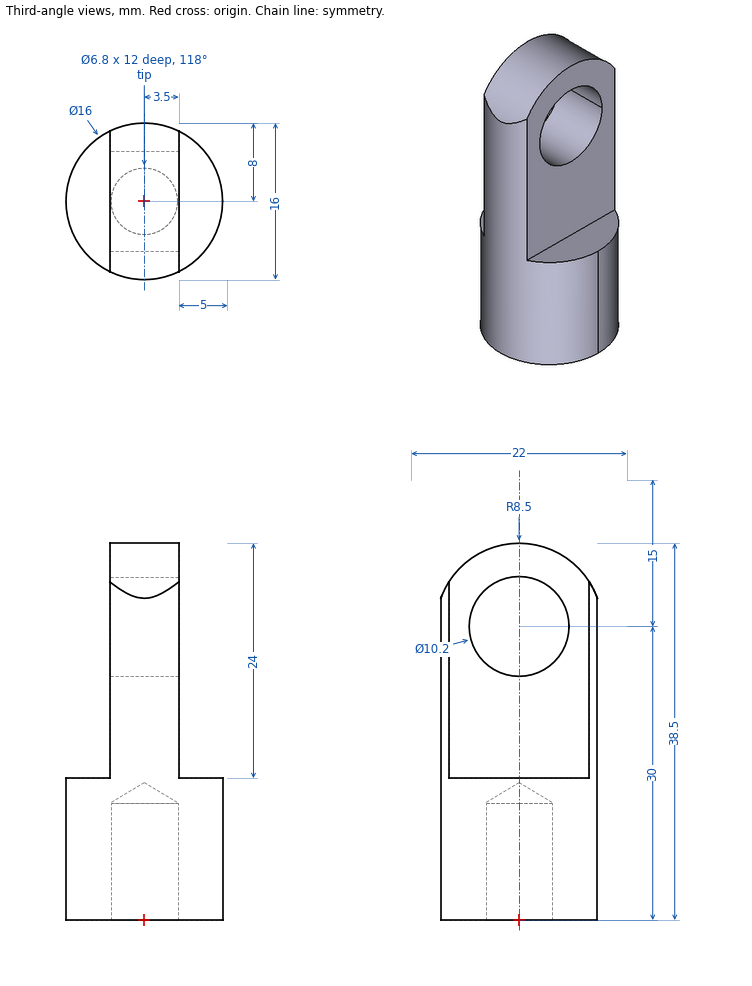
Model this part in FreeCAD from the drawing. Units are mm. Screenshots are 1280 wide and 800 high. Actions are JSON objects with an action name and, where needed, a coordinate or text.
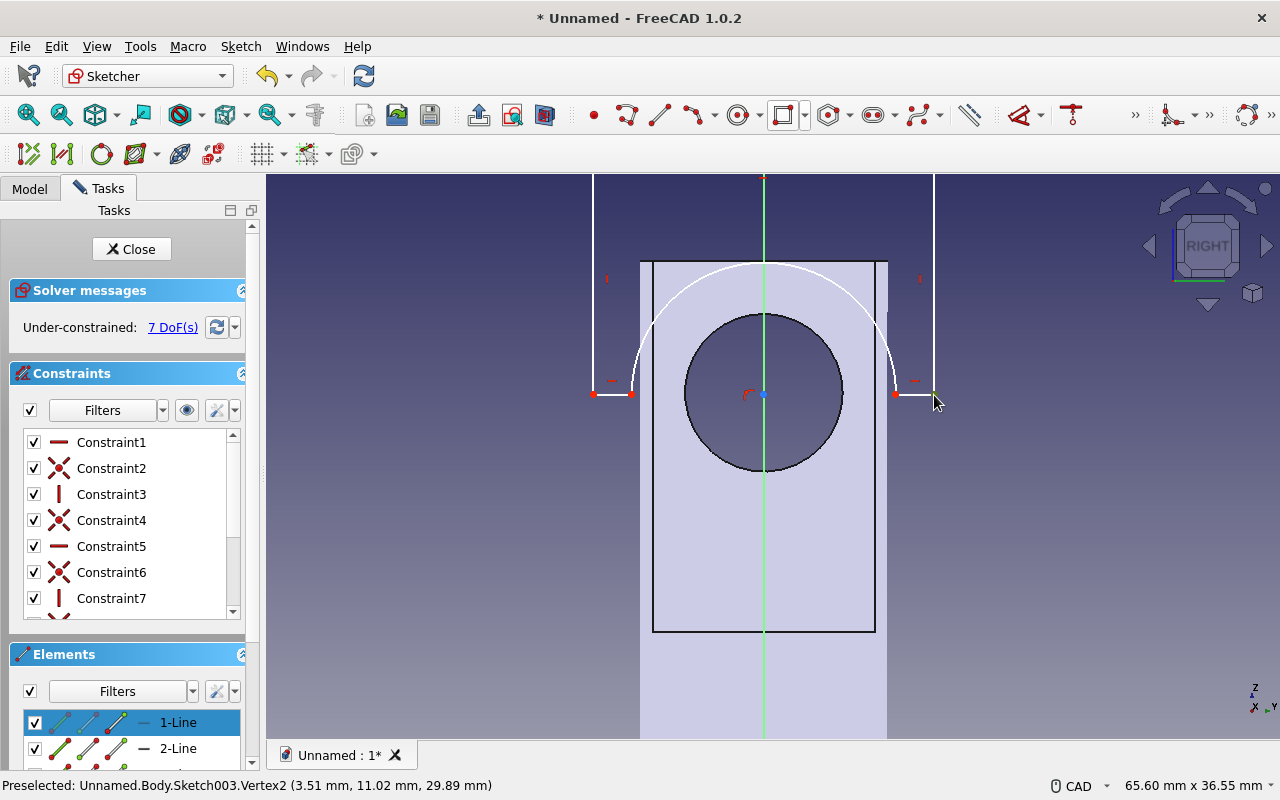
{"action": "left_click", "coordinate": [593, 395]}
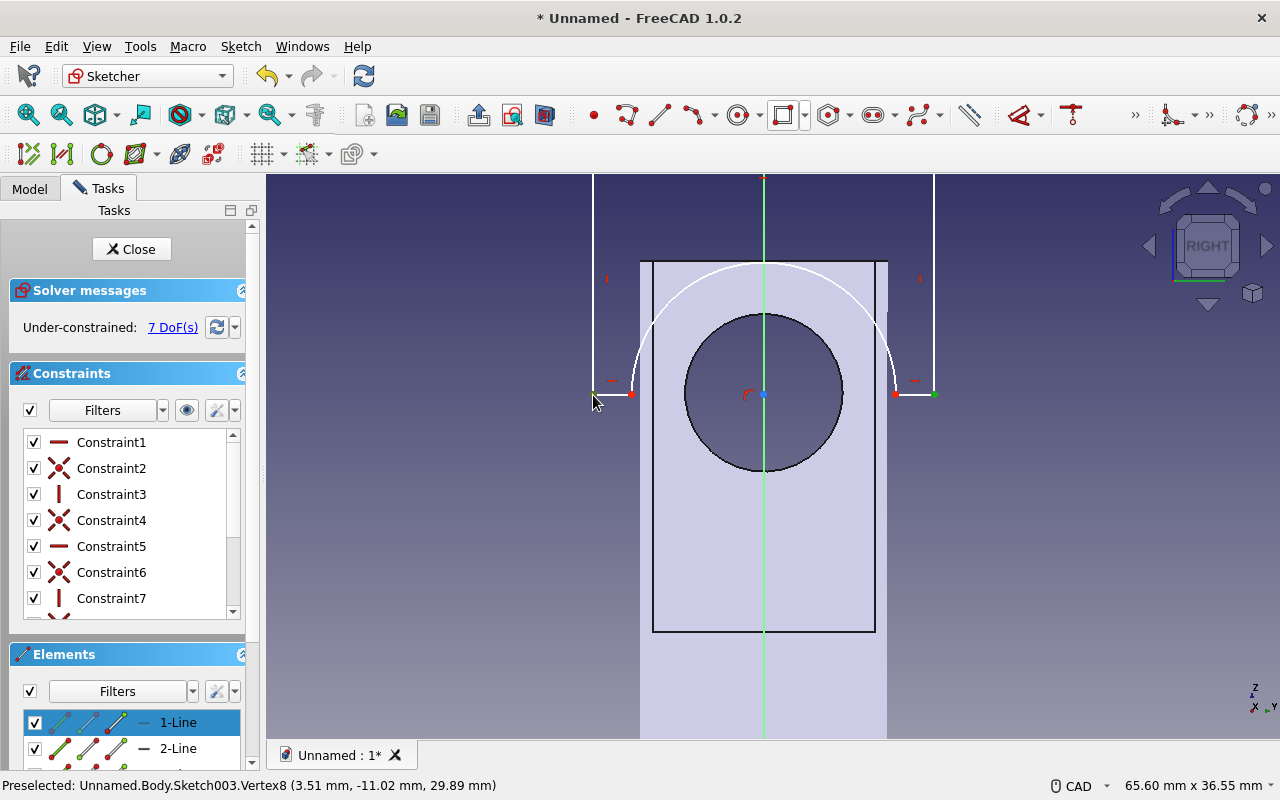
{"action": "left_click", "coordinate": [764, 675]}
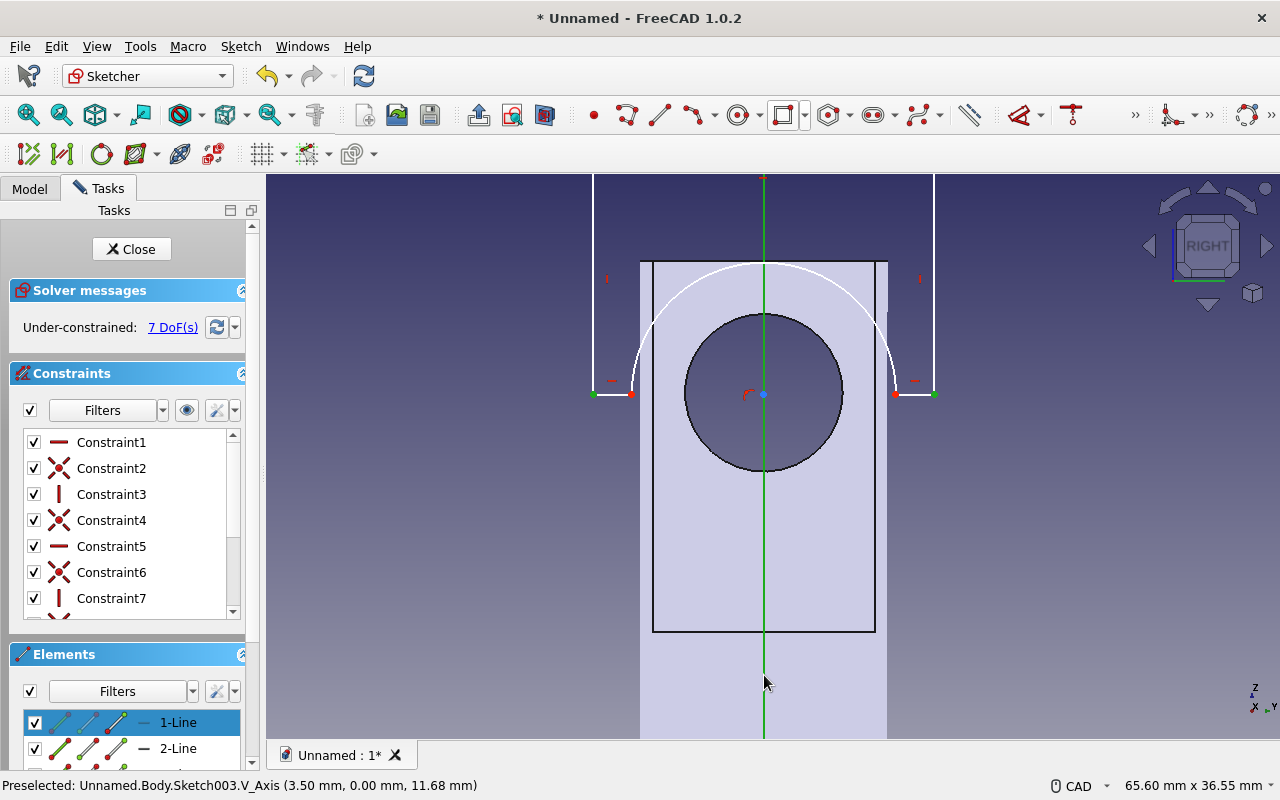
{"action": "key", "text": "s"}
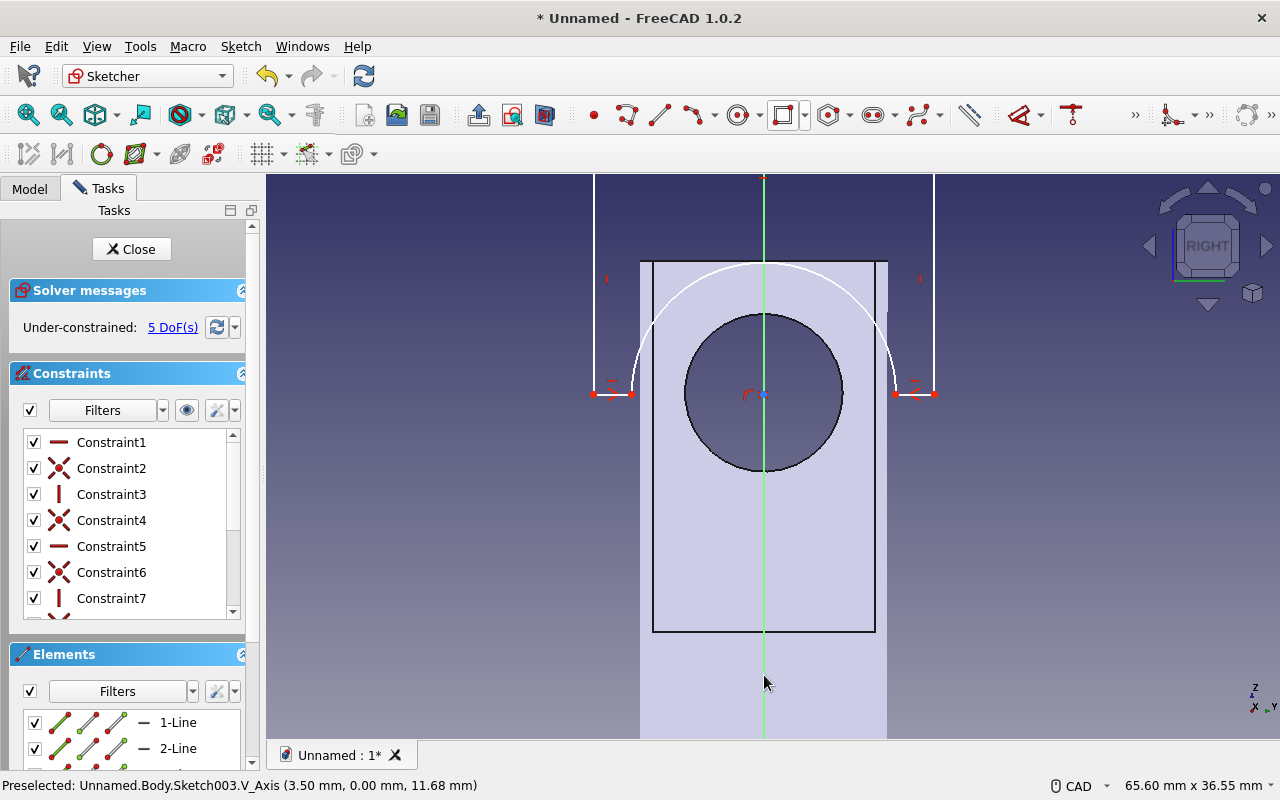
{"action": "key", "text": "d"}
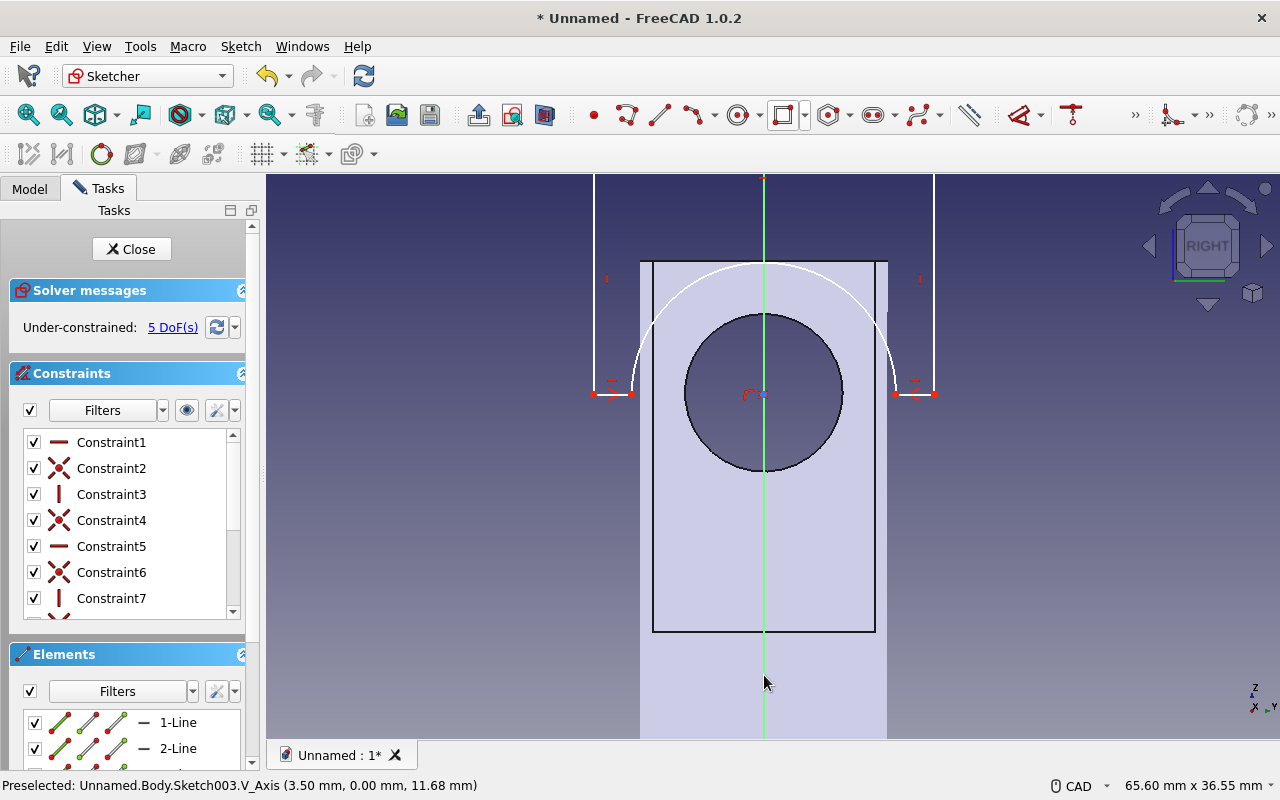
{"action": "left_click", "coordinate": [841, 288]}
{"action": "left_click", "coordinate": [860, 262]}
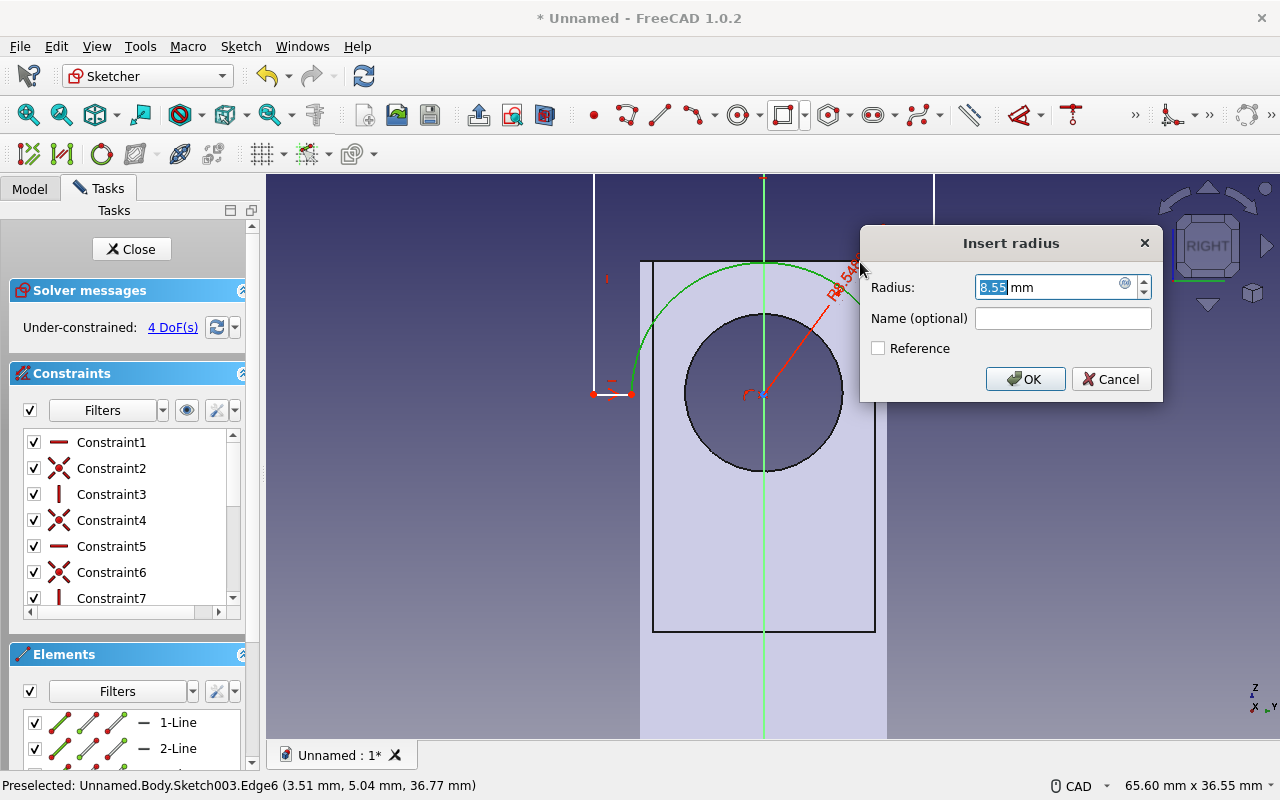
{"action": "type", "text": "8.5"}
{"action": "key", "text": "Return"}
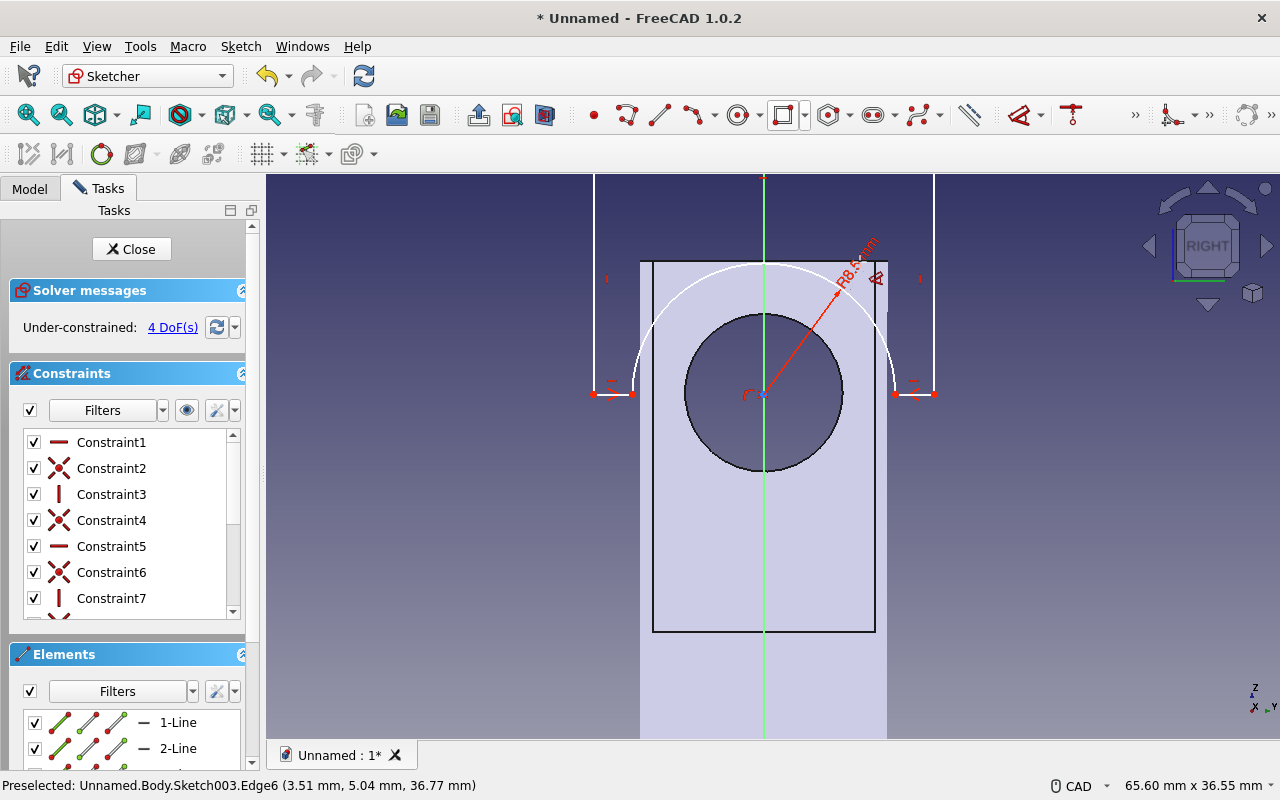
{"action": "left_click", "coordinate": [934, 325]}
{"action": "left_click", "coordinate": [968, 298]}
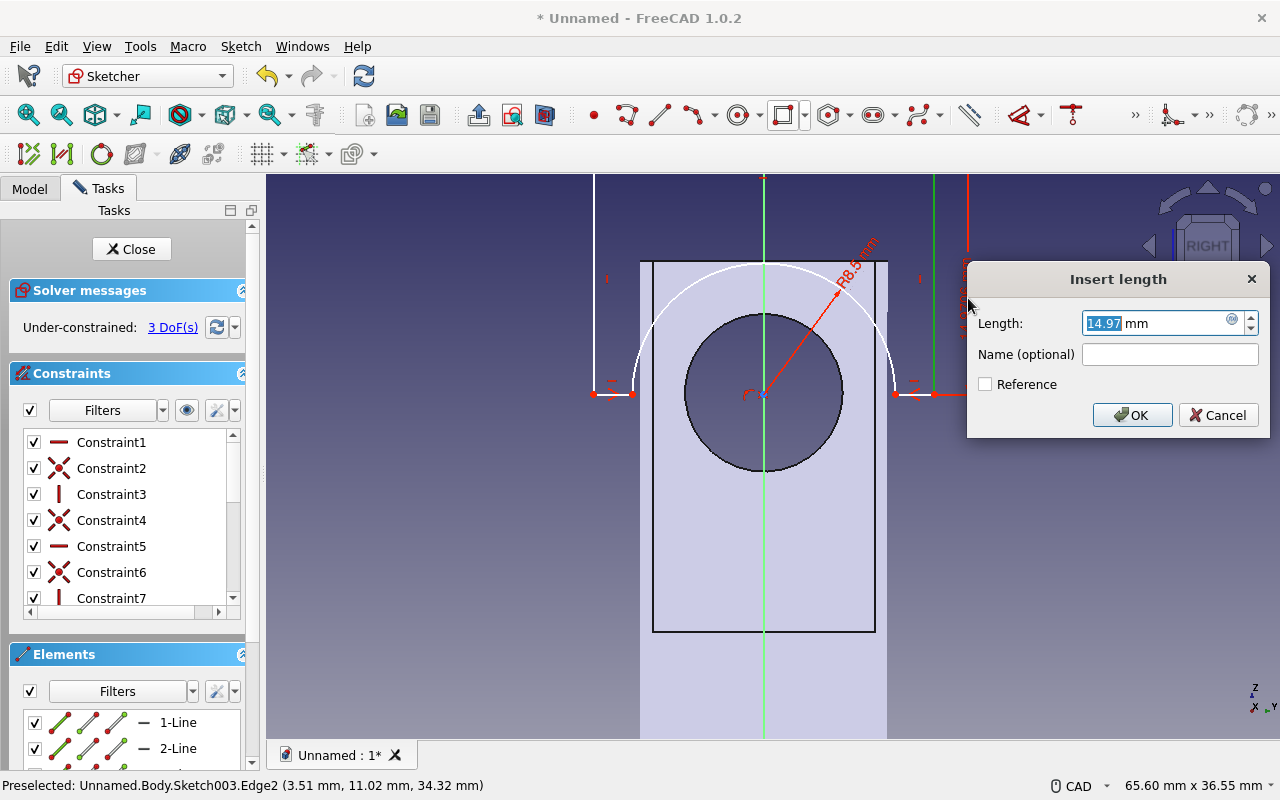
{"action": "type", "text": "15"}
{"action": "key", "text": "Return"}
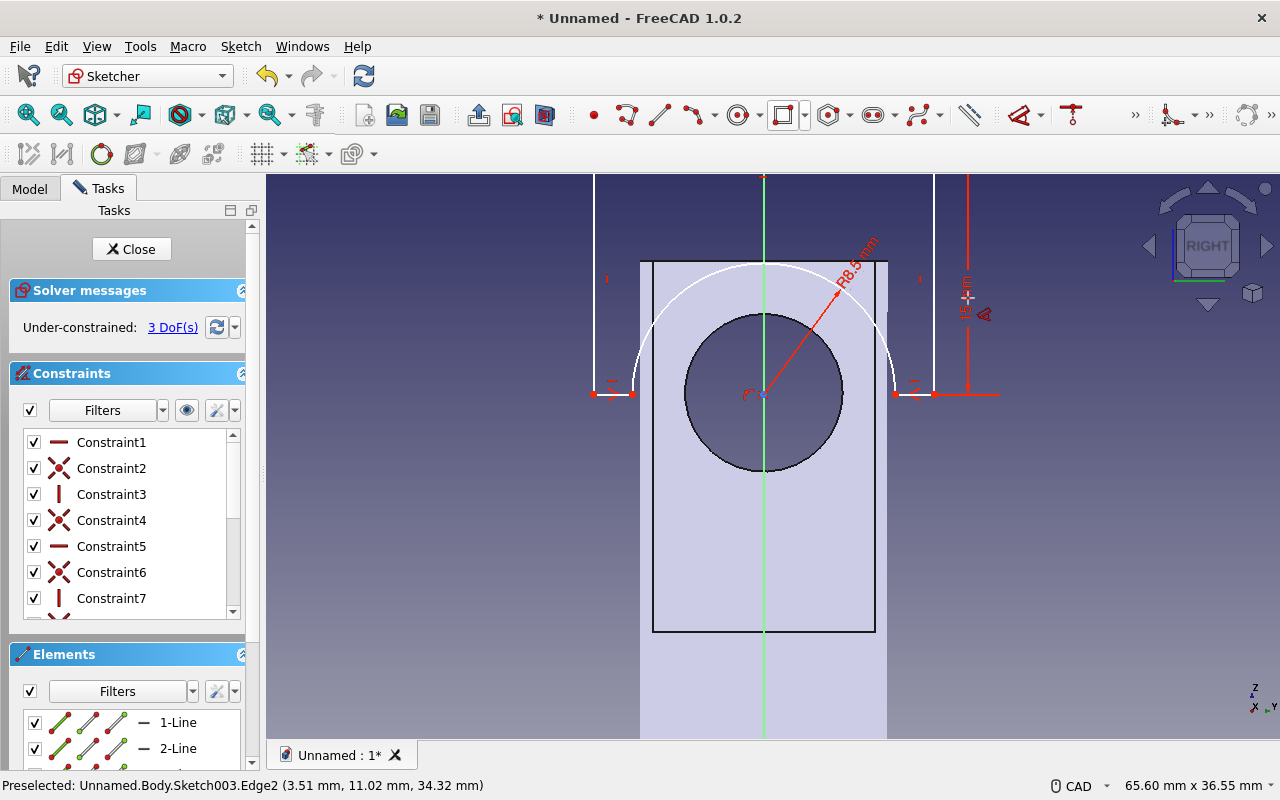
{"action": "scroll", "coordinate": [632, 393], "scroll_direction": "down", "scroll_amount": 3}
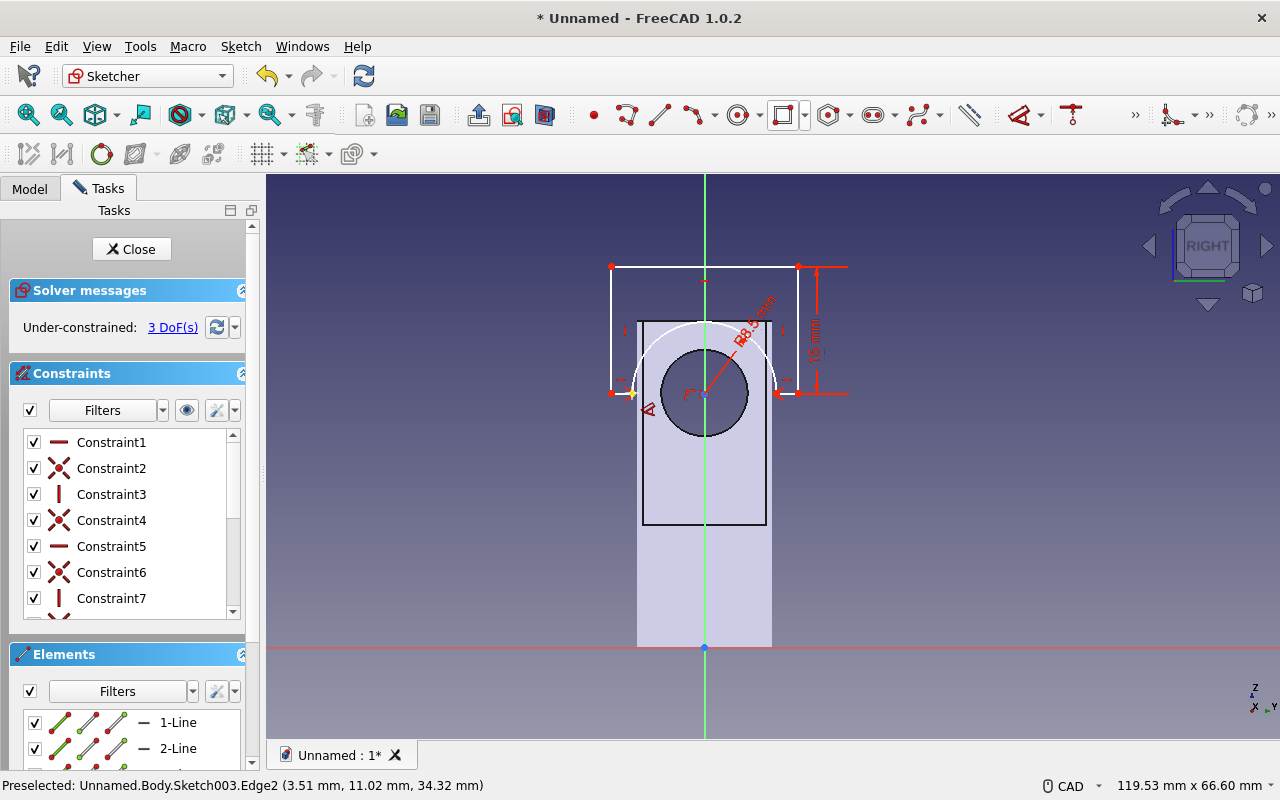
{"action": "left_click", "coordinate": [742, 267]}
{"action": "left_click", "coordinate": [662, 233]}